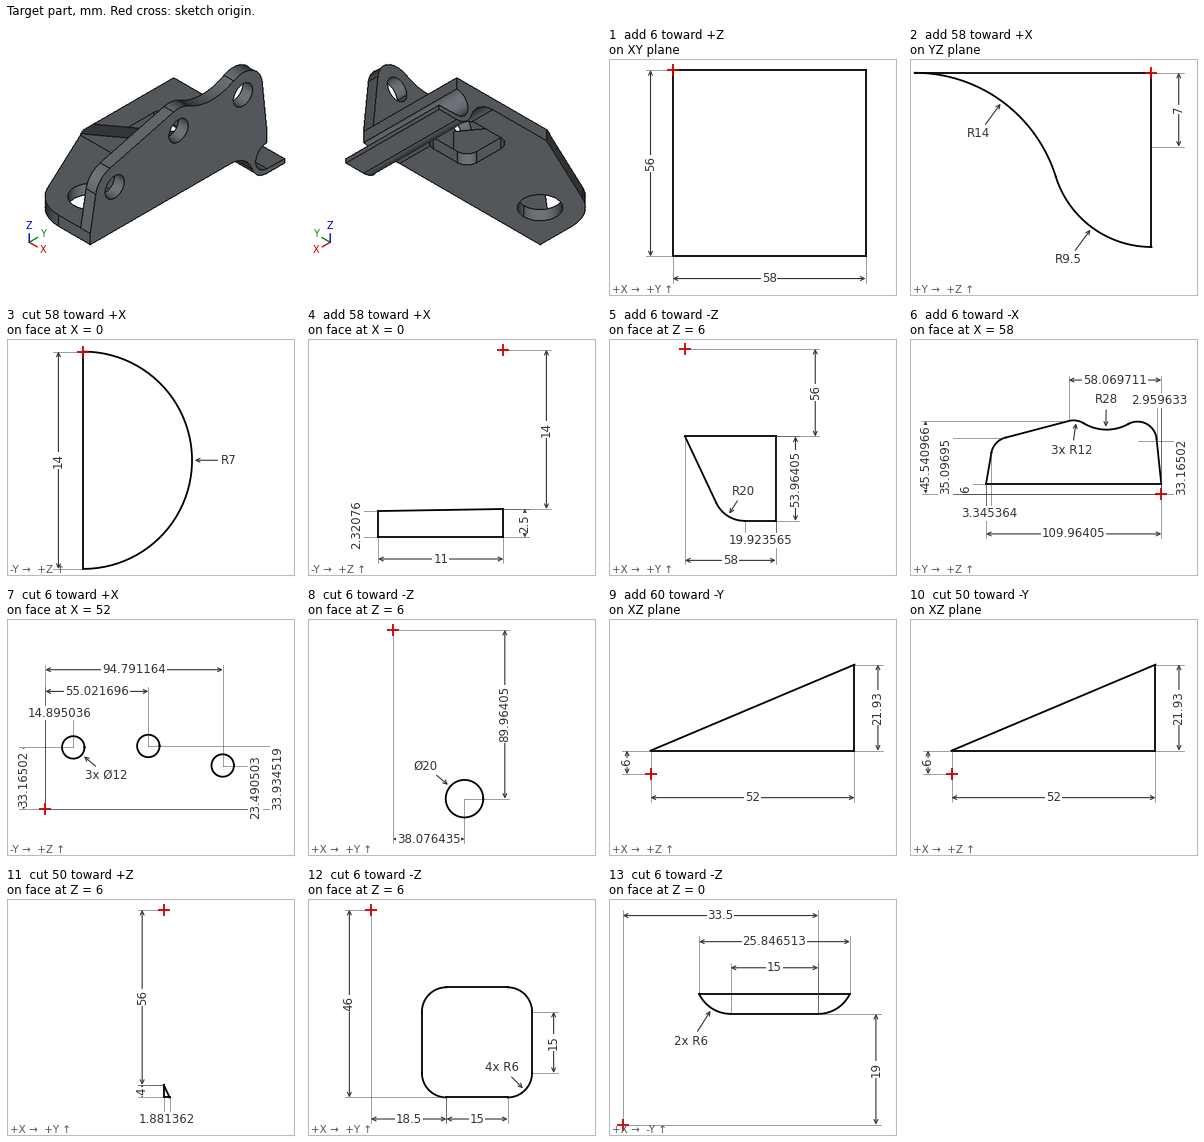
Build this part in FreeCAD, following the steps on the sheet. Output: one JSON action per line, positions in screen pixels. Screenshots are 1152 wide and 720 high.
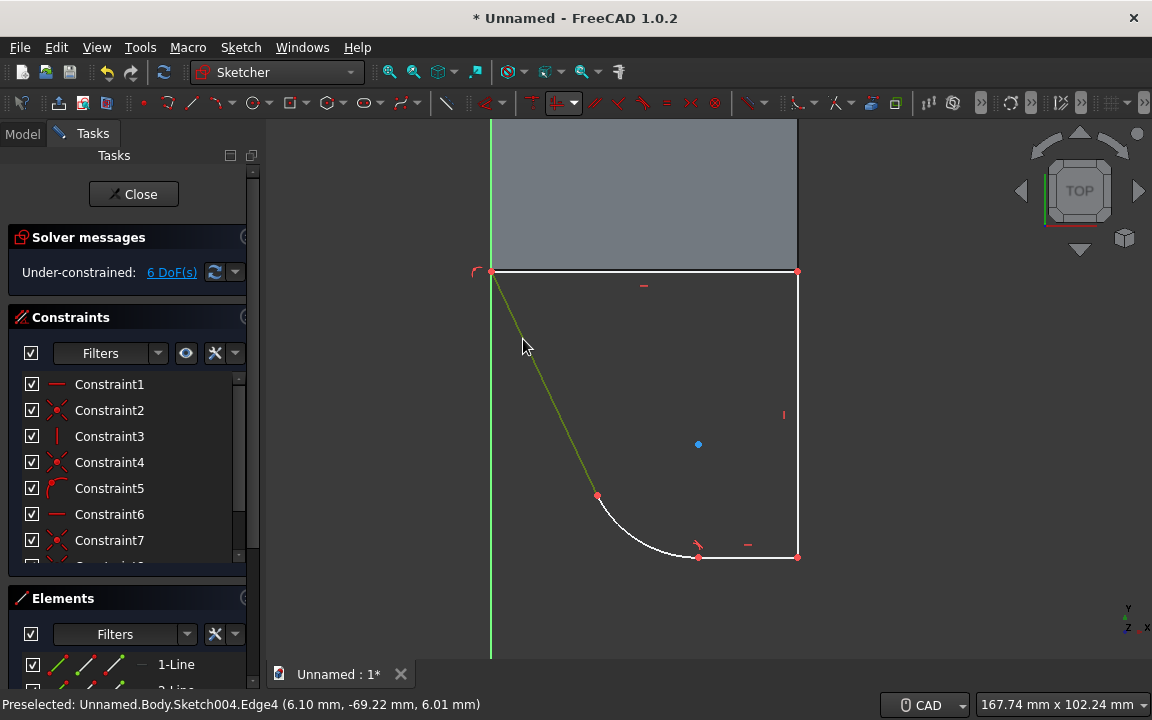
{"action": "left_click", "coordinate": [619, 526]}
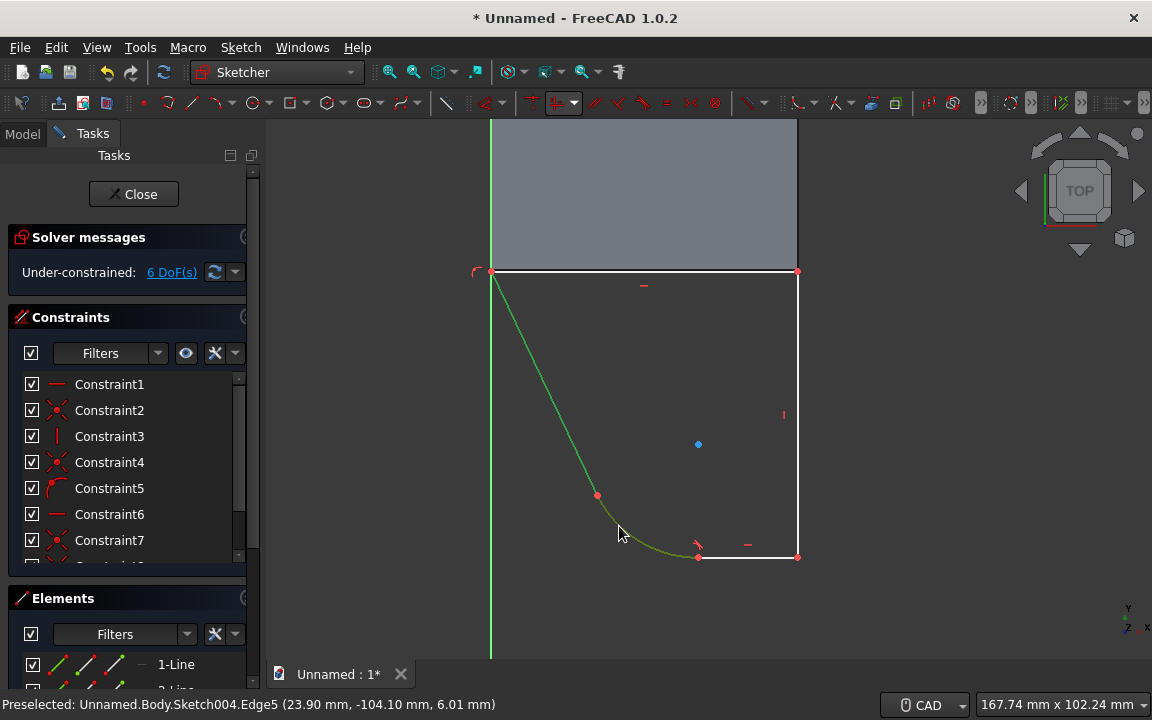
{"action": "left_click", "coordinate": [644, 104]}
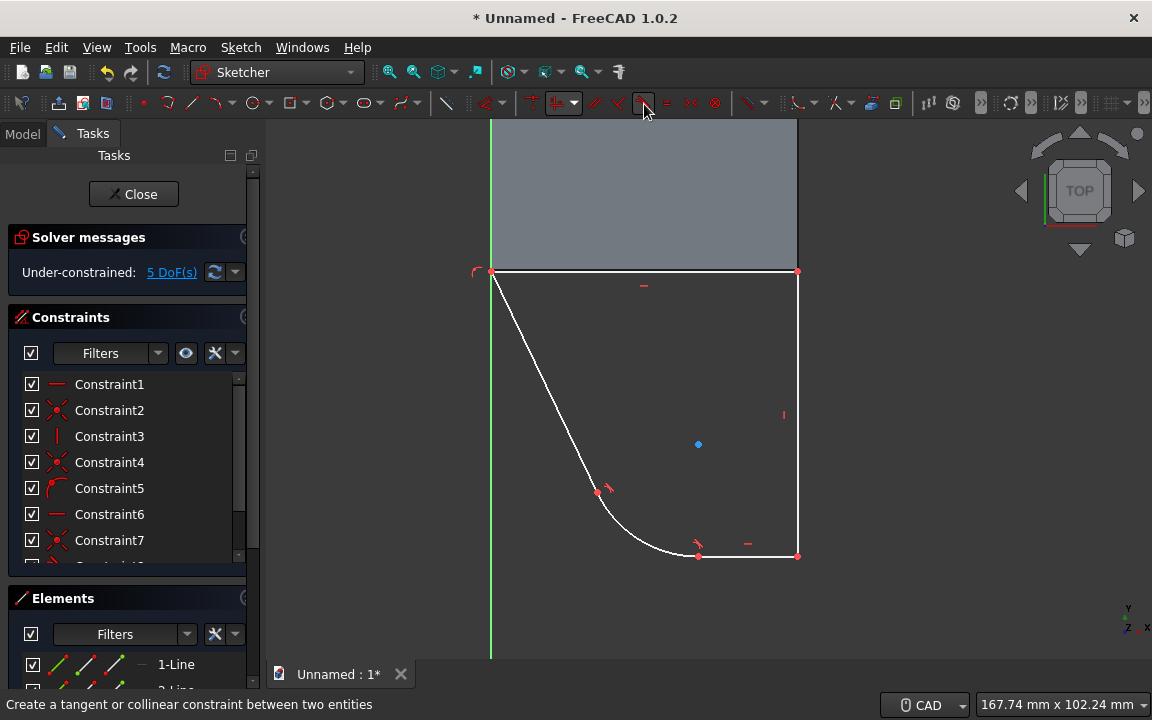
{"action": "left_click", "coordinate": [486, 104]}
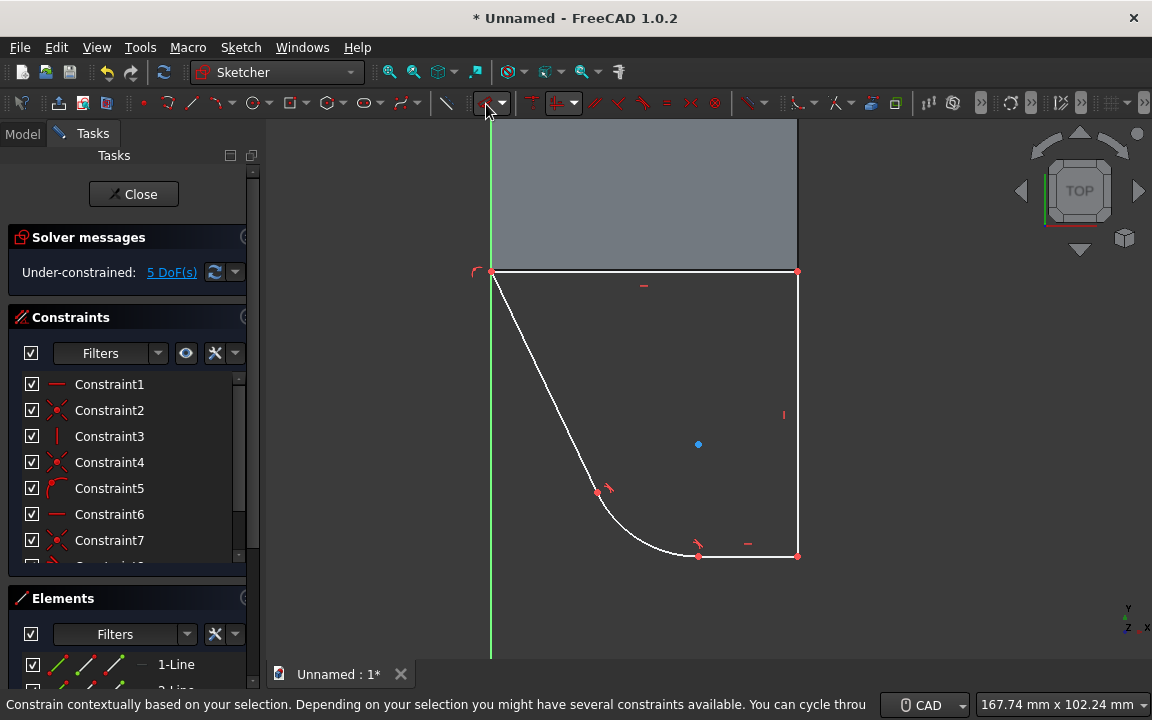
{"action": "left_click", "coordinate": [619, 524]}
{"action": "left_click", "coordinate": [596, 547]}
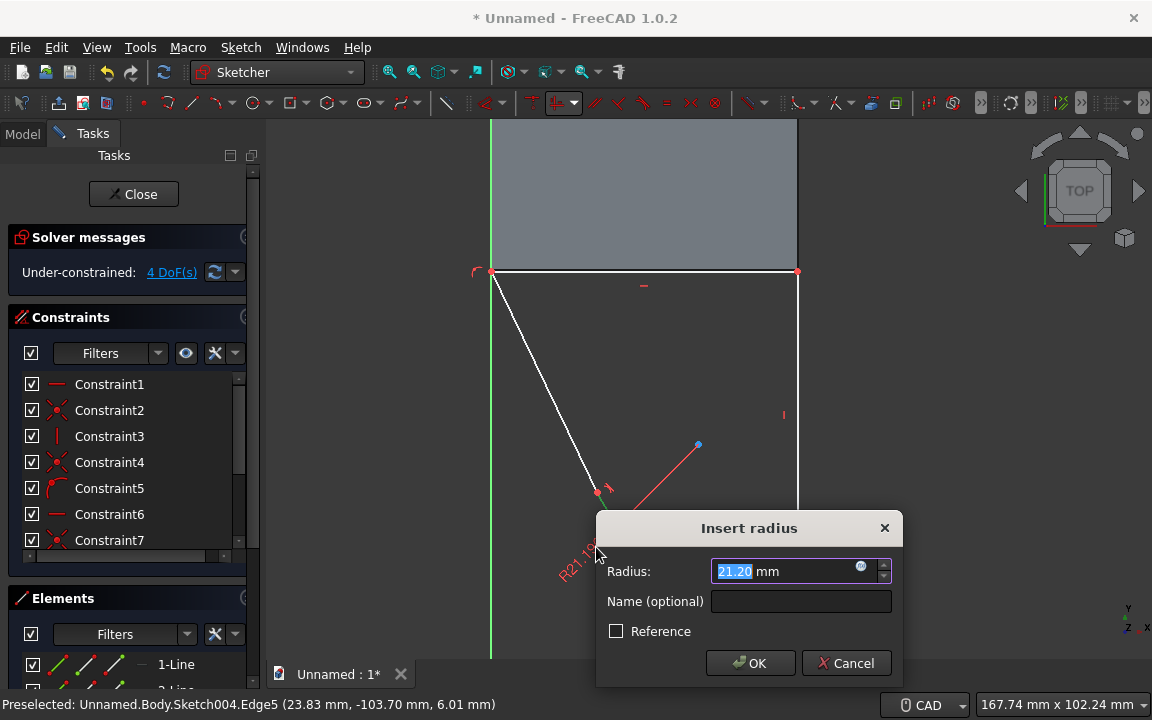
{"action": "type", "text": "20"}
{"action": "key", "text": "Return"}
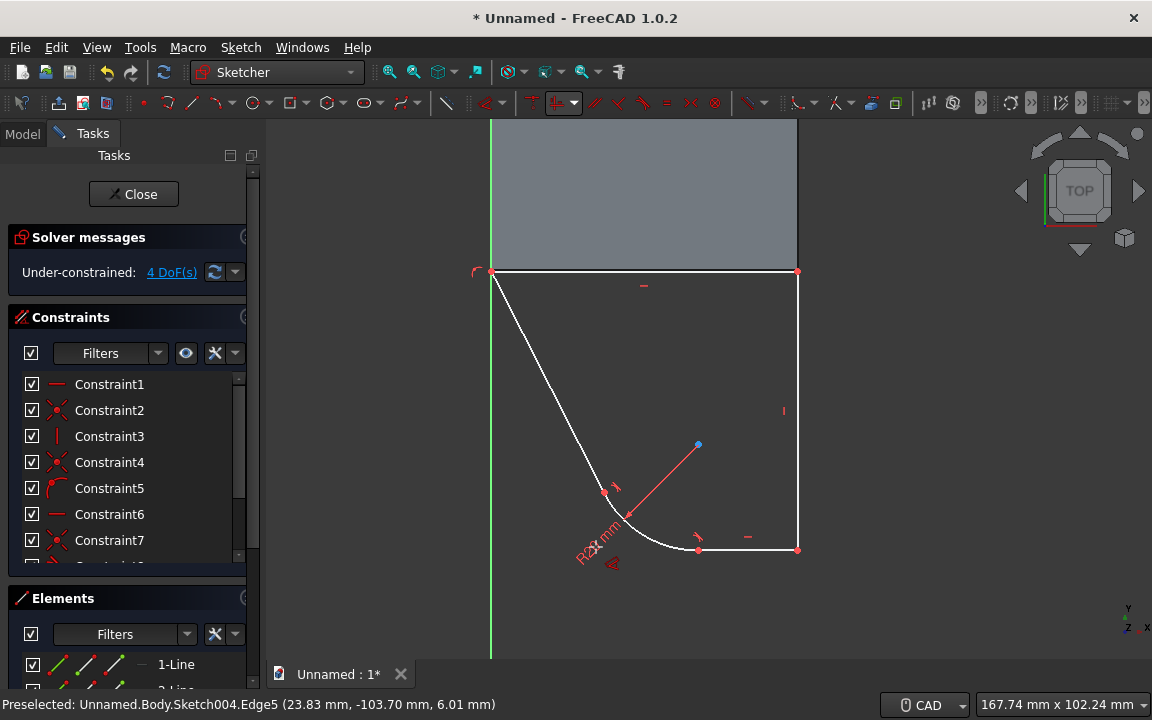
{"action": "left_click", "coordinate": [706, 272]}
{"action": "left_click", "coordinate": [645, 306]}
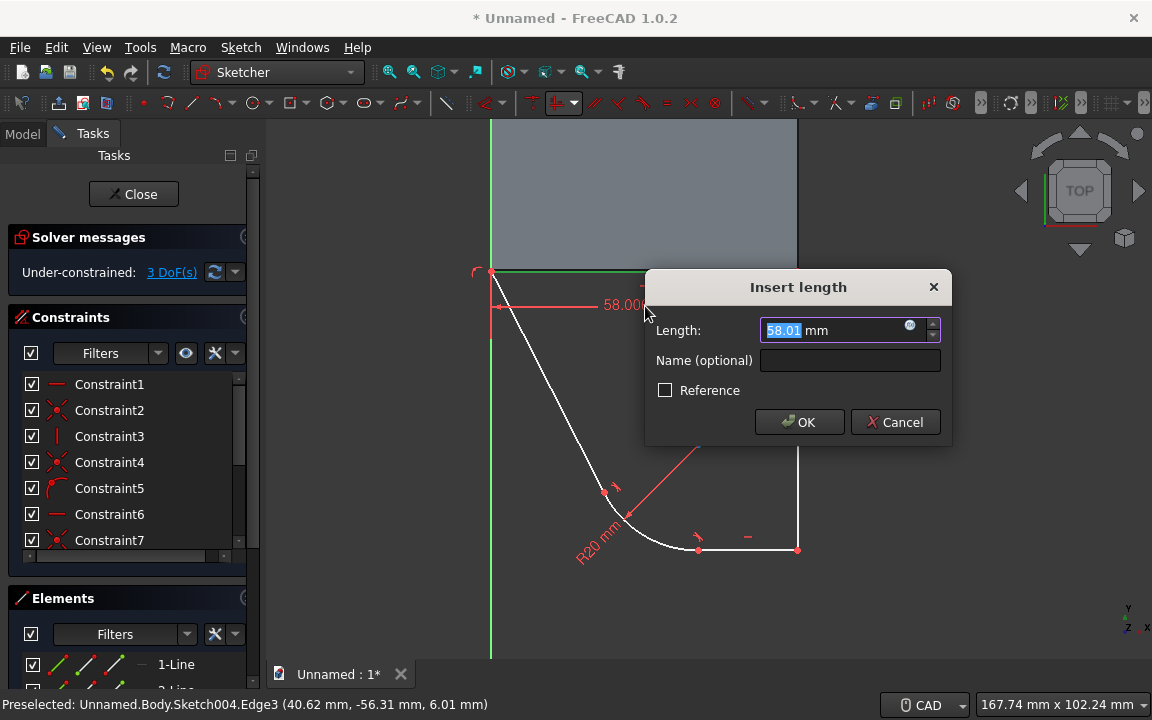
{"action": "type", "text": "58"}
{"action": "key", "text": "Return"}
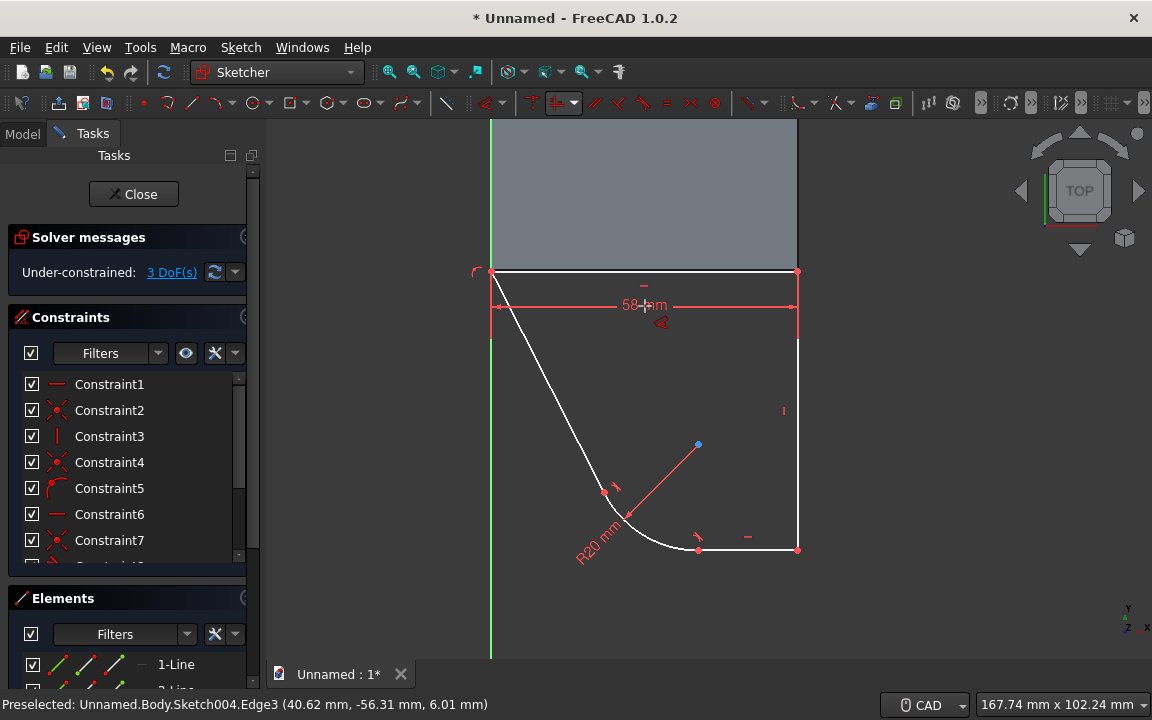
{"action": "left_click", "coordinate": [798, 272]}
{"action": "left_click", "coordinate": [832, 209]}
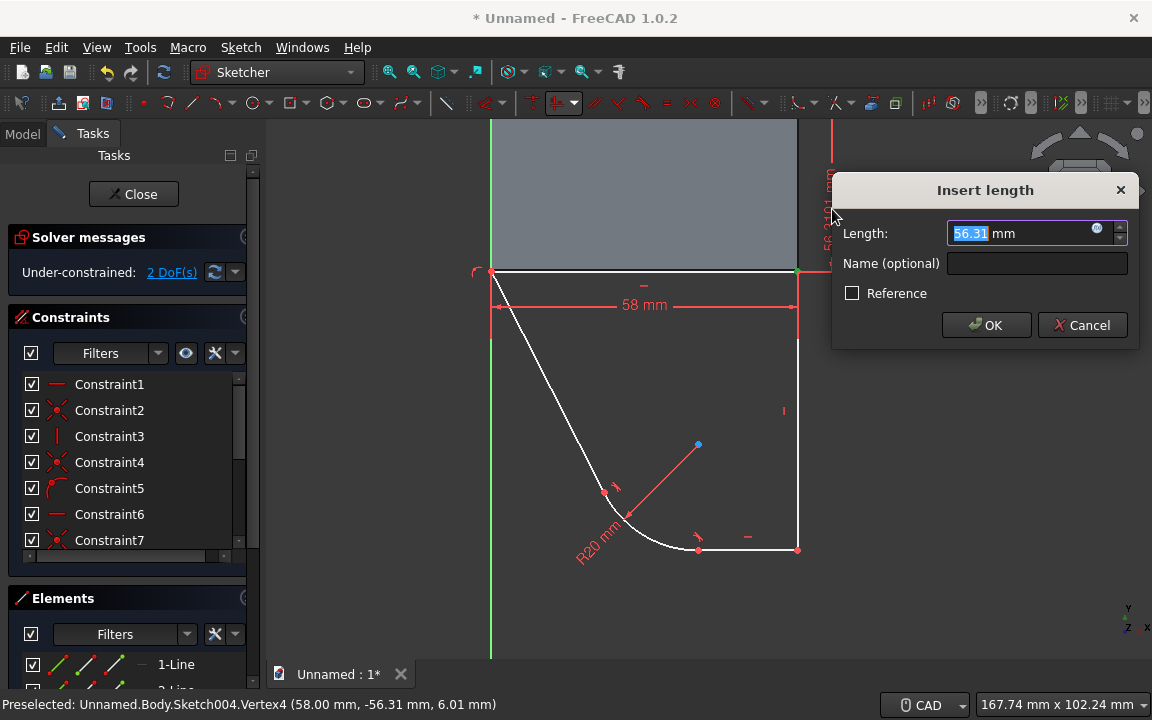
{"action": "type", "text": "56"}
{"action": "key", "text": "Return"}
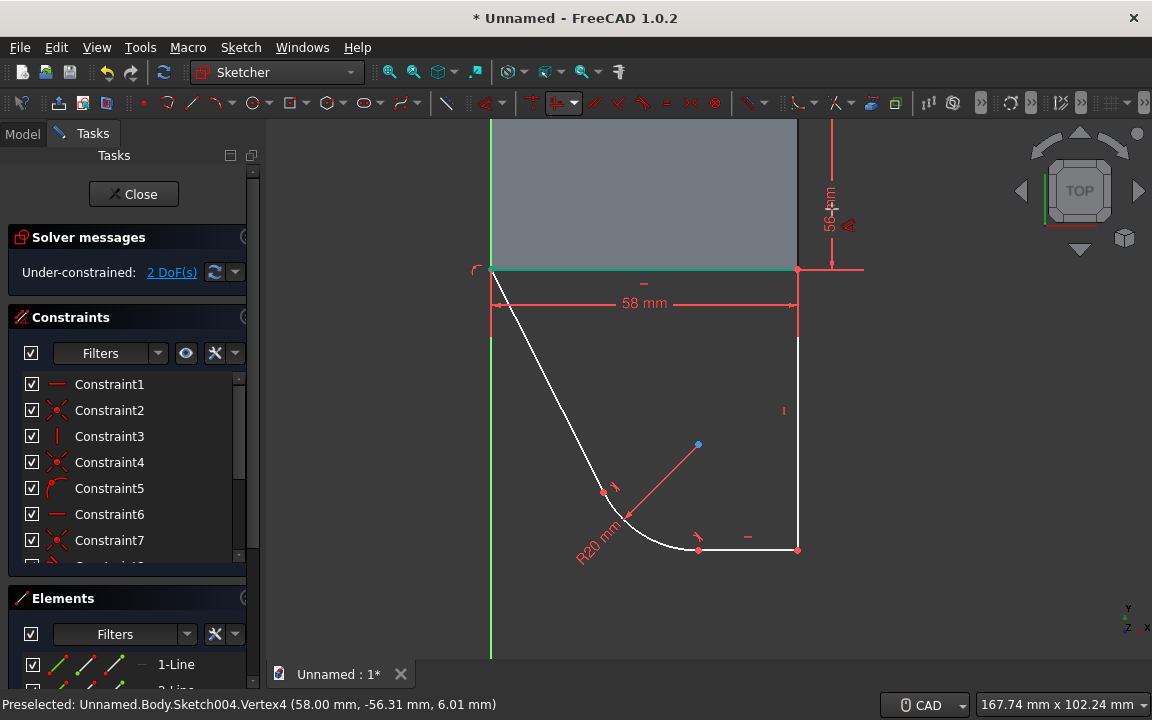
{"action": "left_click", "coordinate": [798, 466]}
{"action": "left_click", "coordinate": [832, 410]}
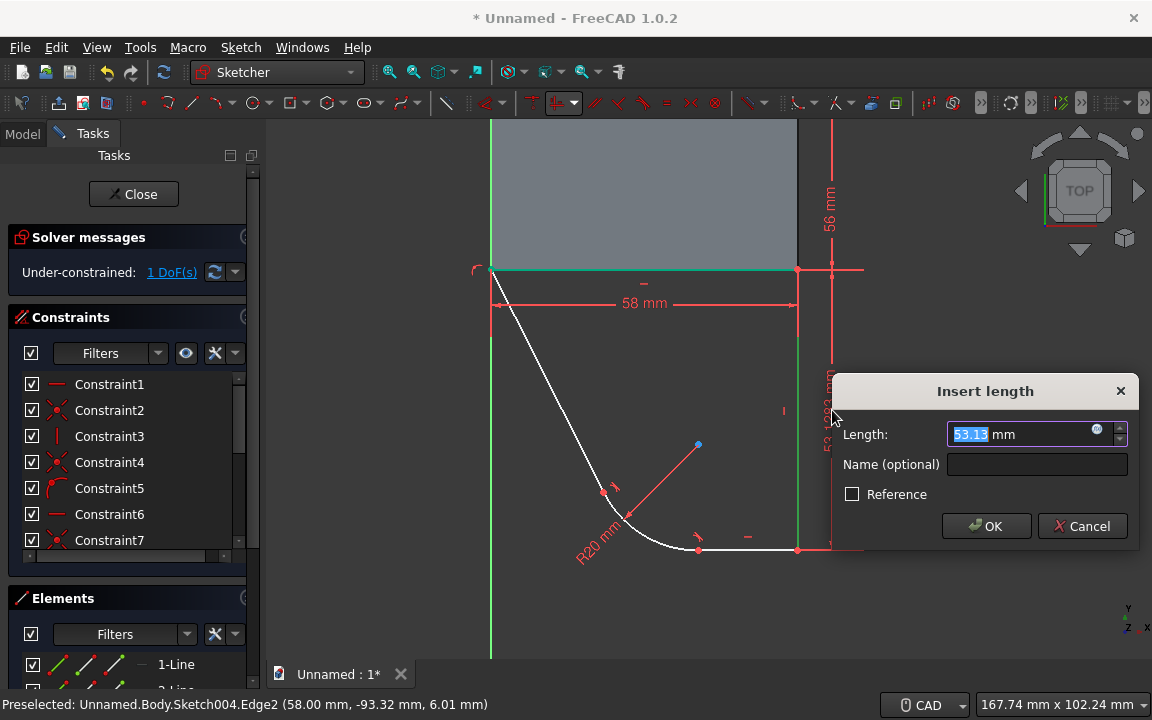
{"action": "type", "text": "53.96405"}
{"action": "key", "text": "Return"}